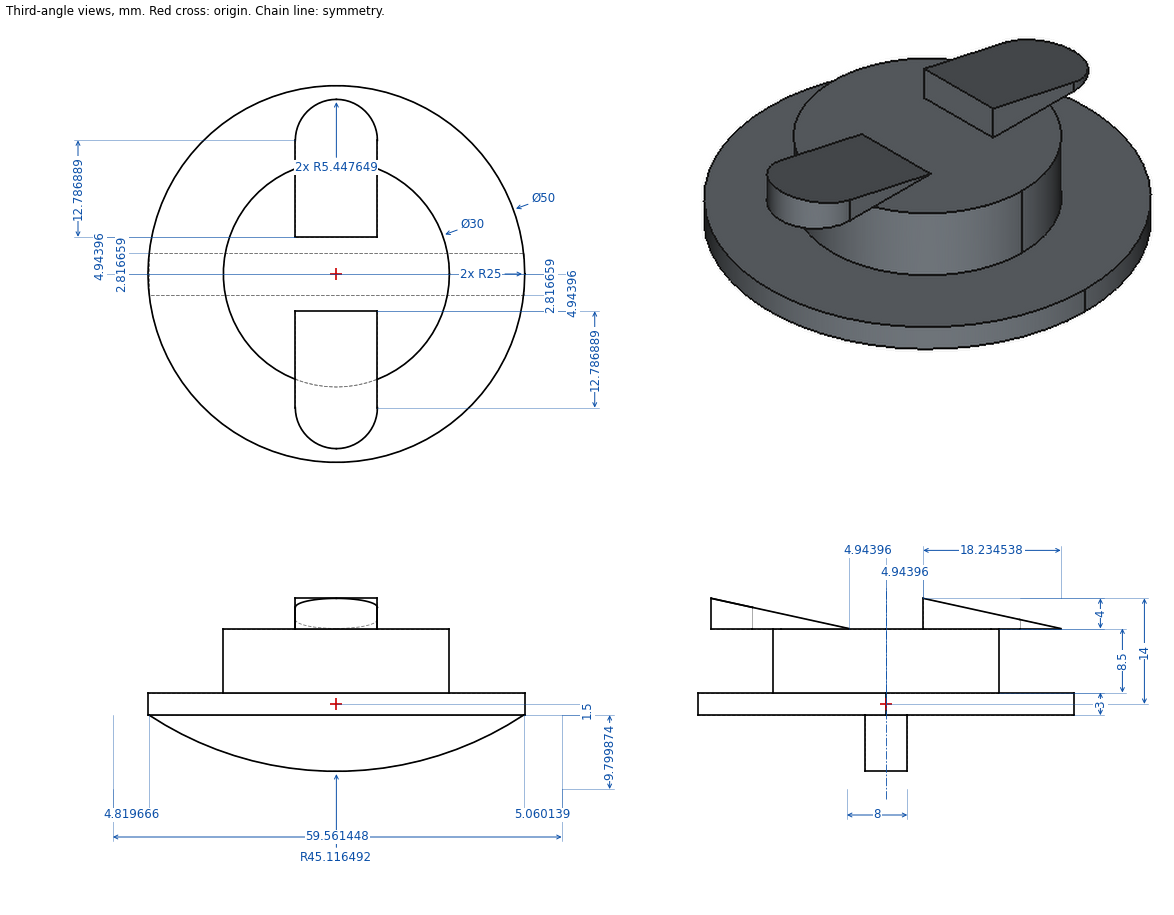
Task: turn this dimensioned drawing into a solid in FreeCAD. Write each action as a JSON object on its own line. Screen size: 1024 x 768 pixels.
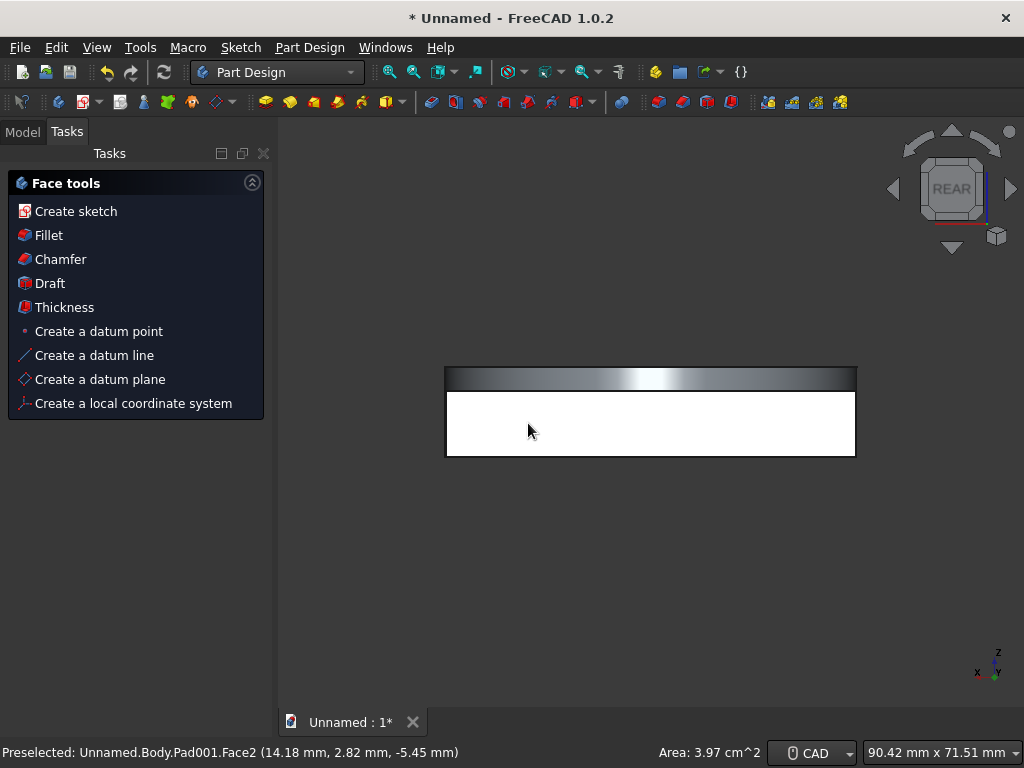
{"action": "left_click", "coordinate": [84, 102]}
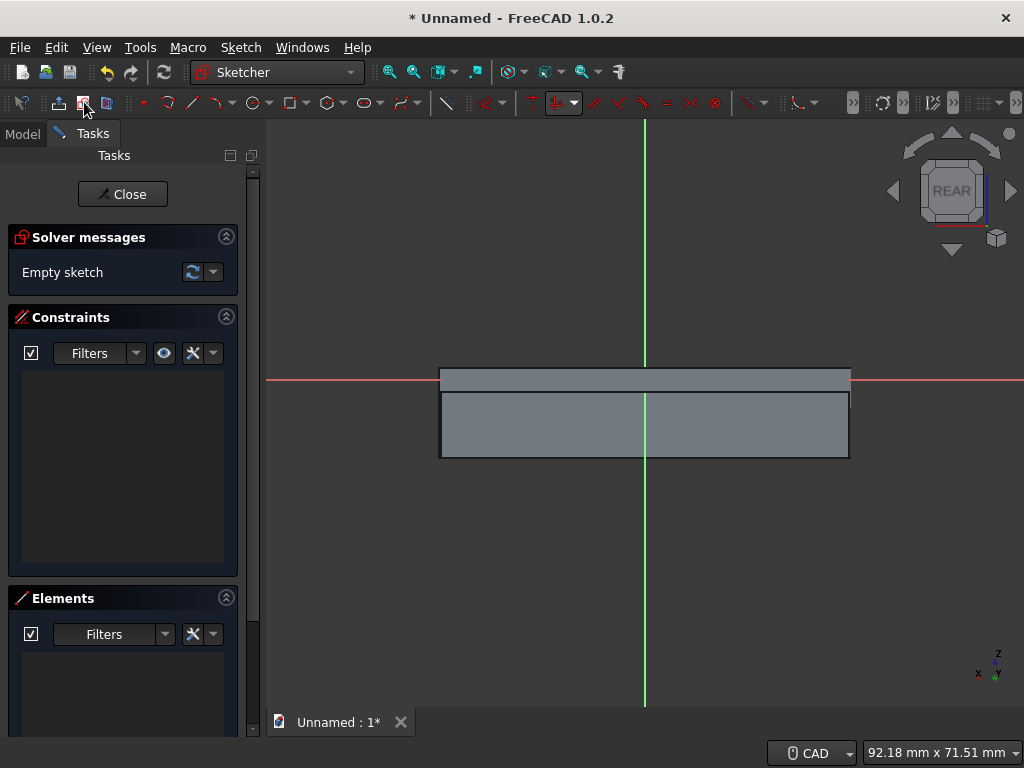
{"action": "left_click", "coordinate": [108, 104]}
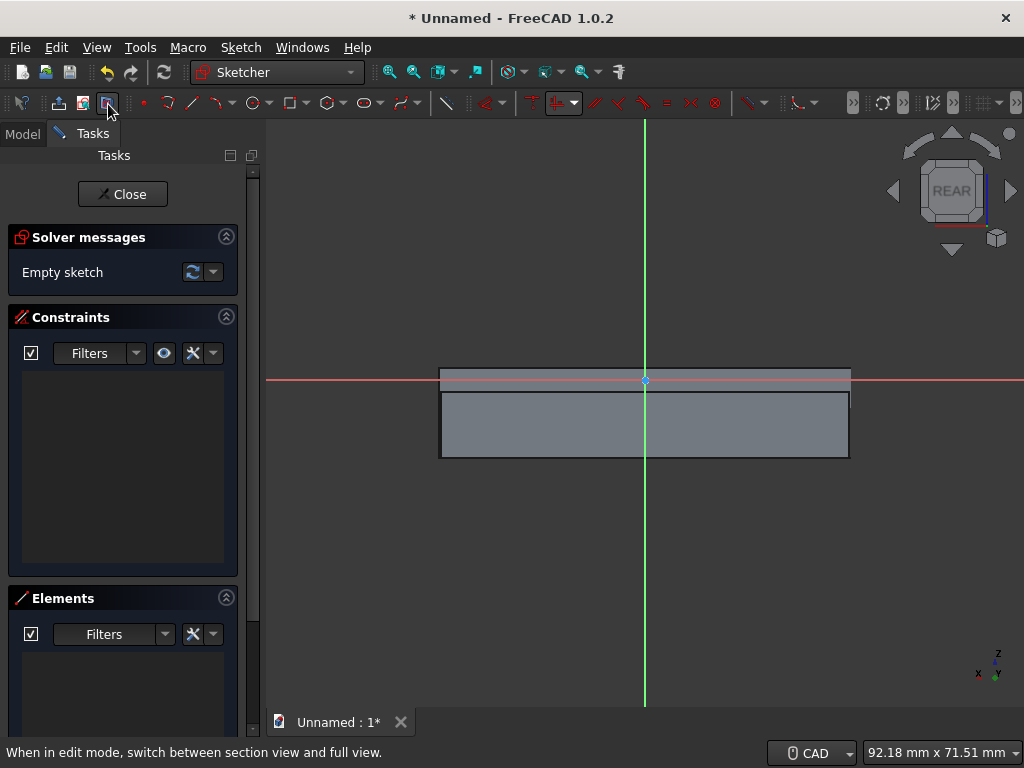
{"action": "scroll", "coordinate": [294, 352], "scroll_direction": "down", "scroll_amount": 1}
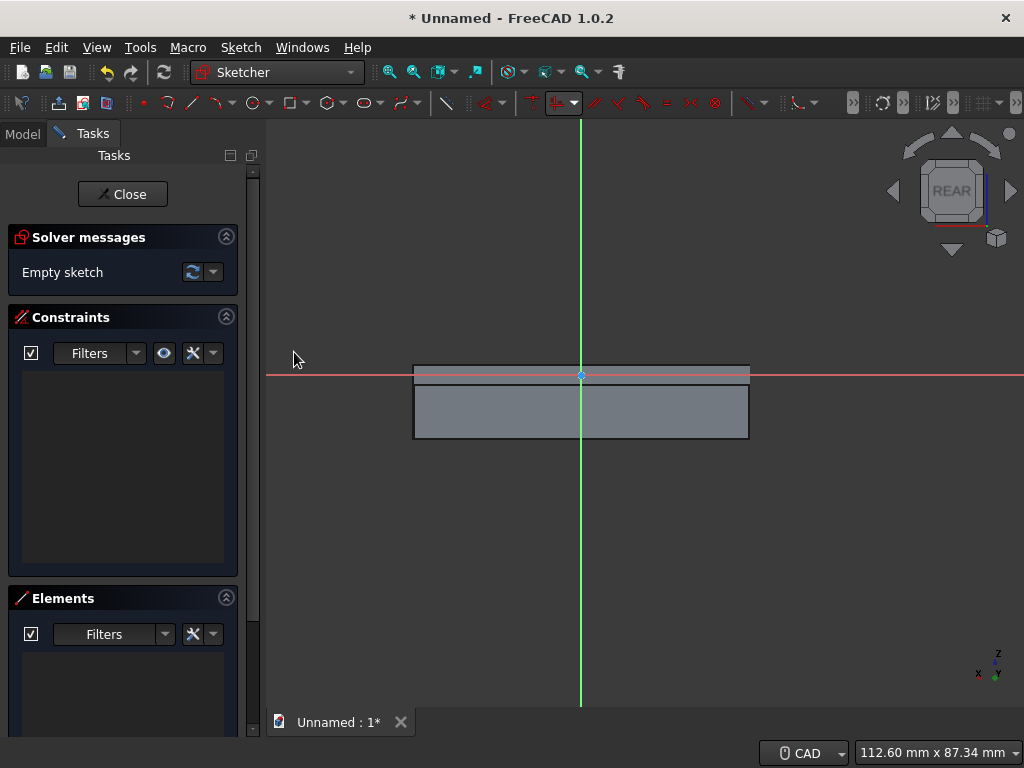
{"action": "left_click", "coordinate": [168, 104]}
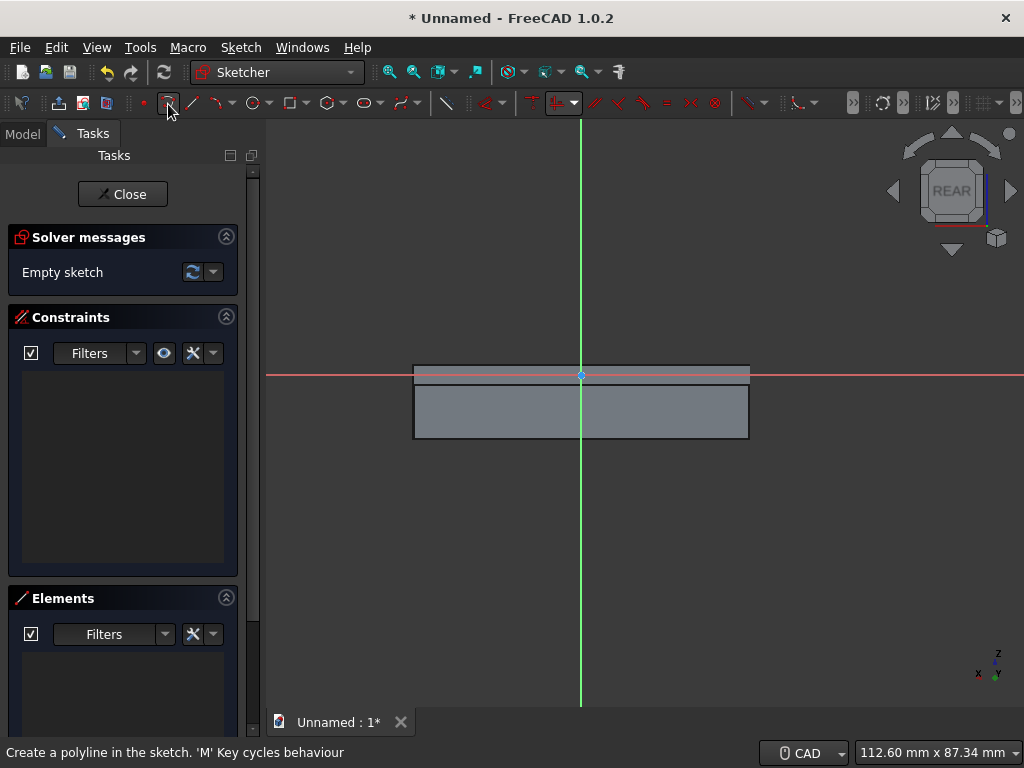
{"action": "scroll", "coordinate": [414, 385], "scroll_direction": "up", "scroll_amount": 3}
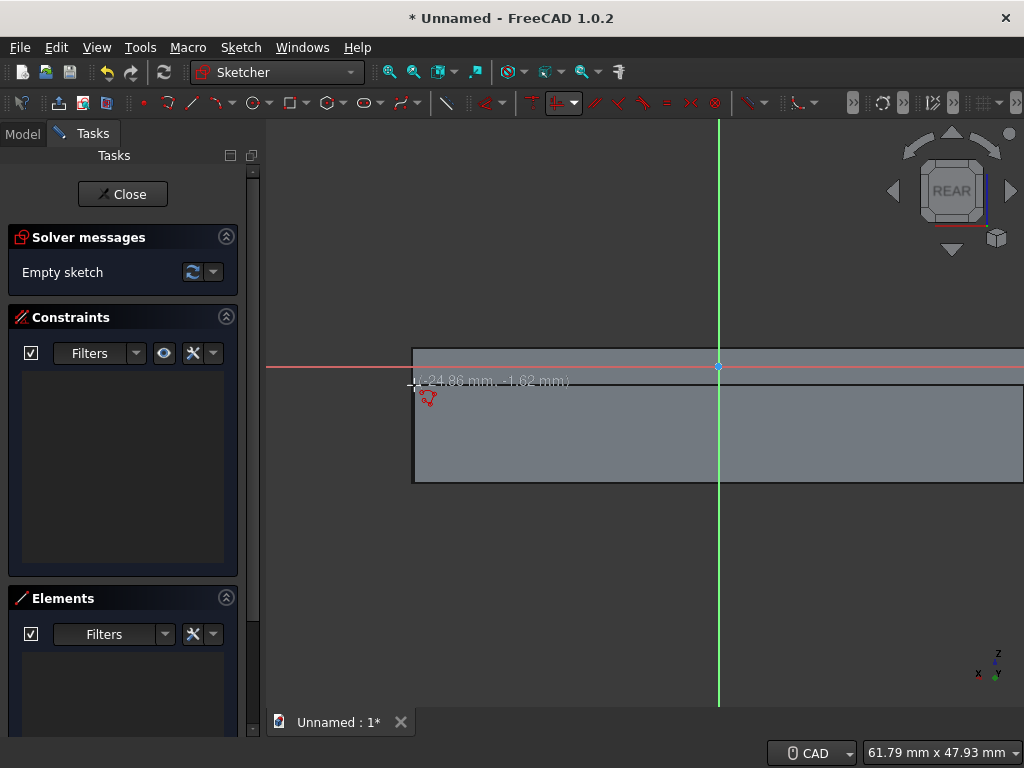
{"action": "left_click", "coordinate": [414, 385]}
{"action": "left_click", "coordinate": [352, 385]}
{"action": "left_click", "coordinate": [352, 505]}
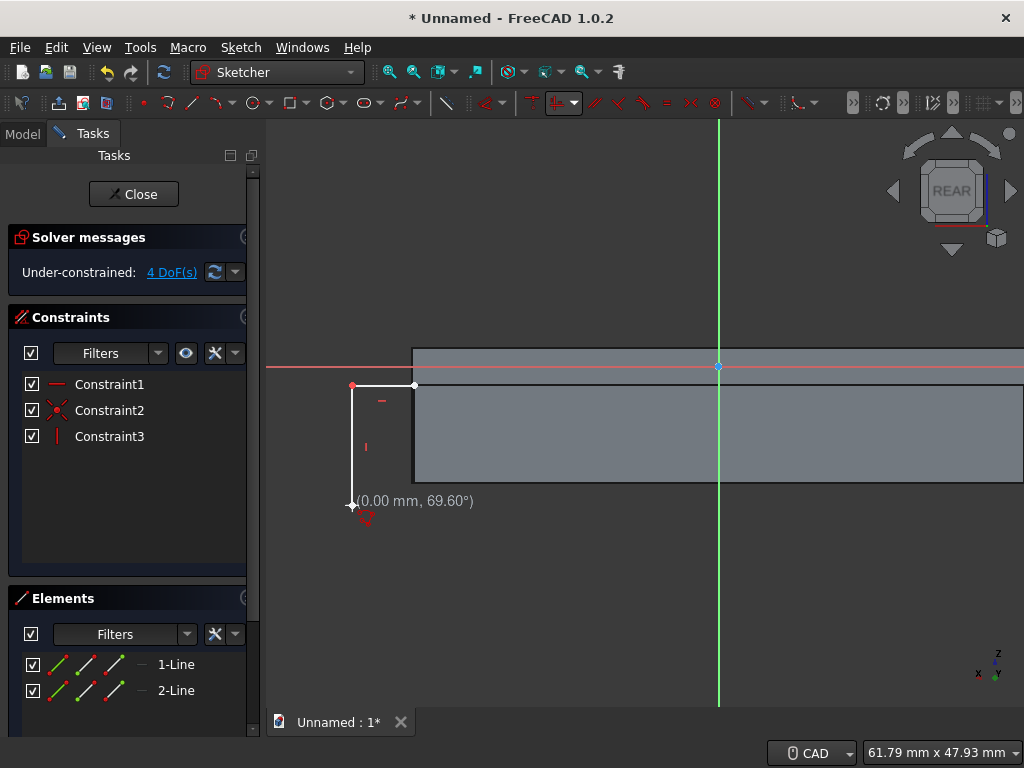
{"action": "scroll", "coordinate": [405, 385], "scroll_direction": "down", "scroll_amount": 3}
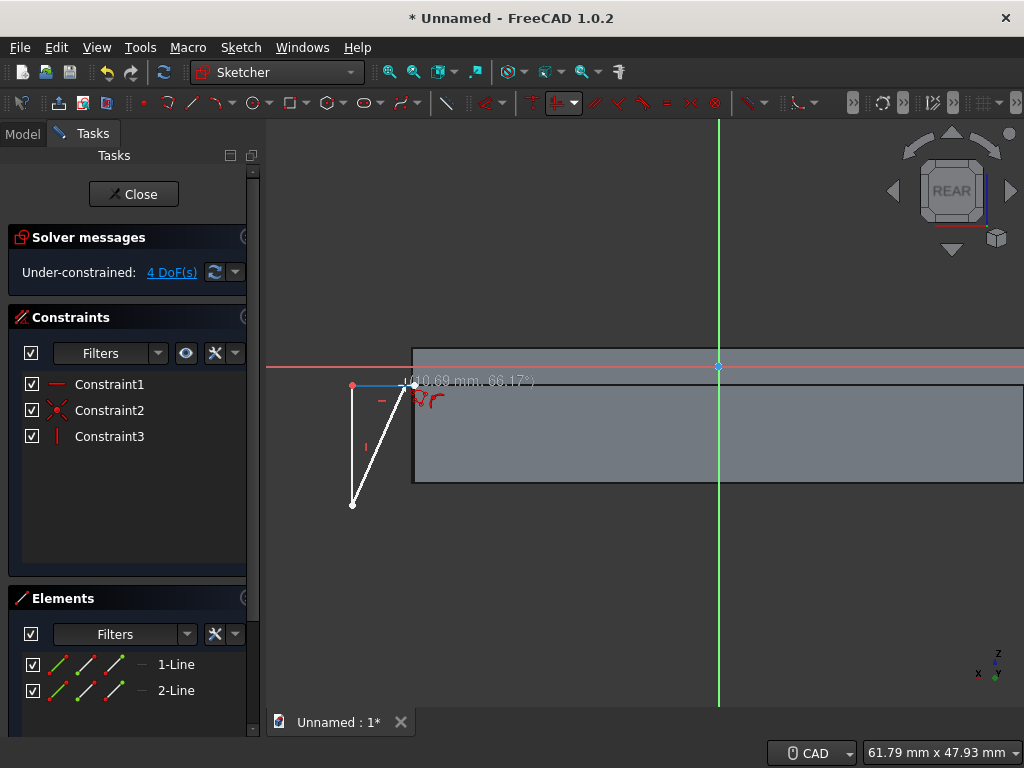
{"action": "left_click", "coordinate": [777, 451]}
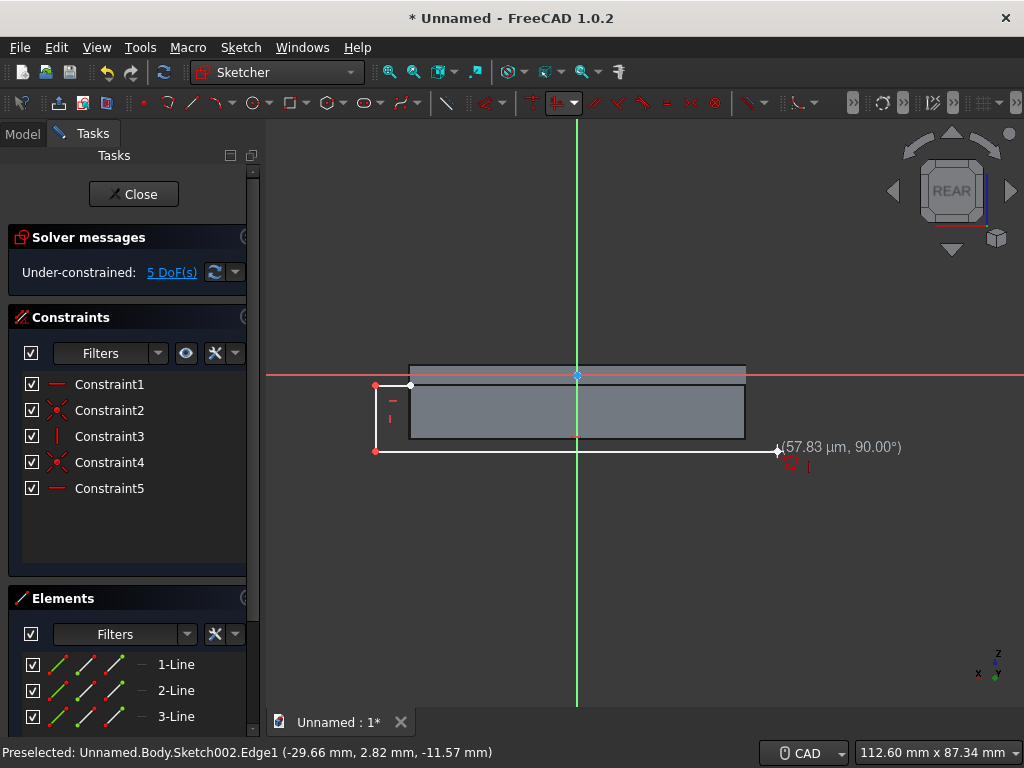
{"action": "scroll", "coordinate": [777, 385], "scroll_direction": "up", "scroll_amount": 3}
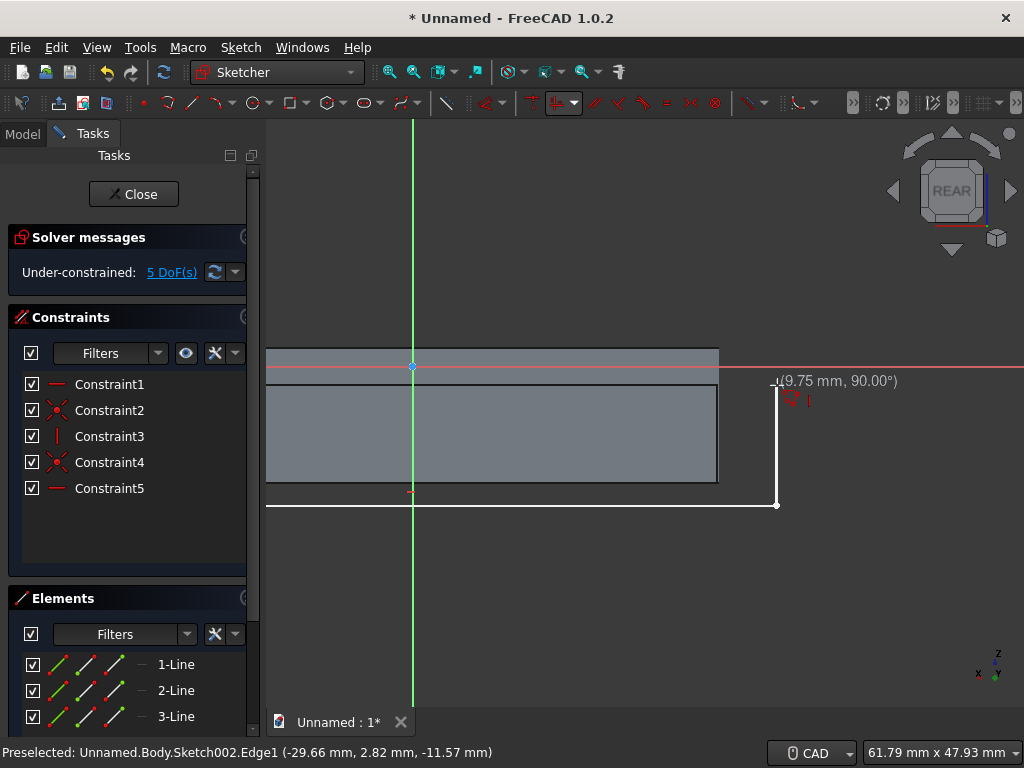
{"action": "left_click", "coordinate": [776, 385]}
{"action": "left_click", "coordinate": [717, 385]}
{"action": "right_click", "coordinate": [717, 385]}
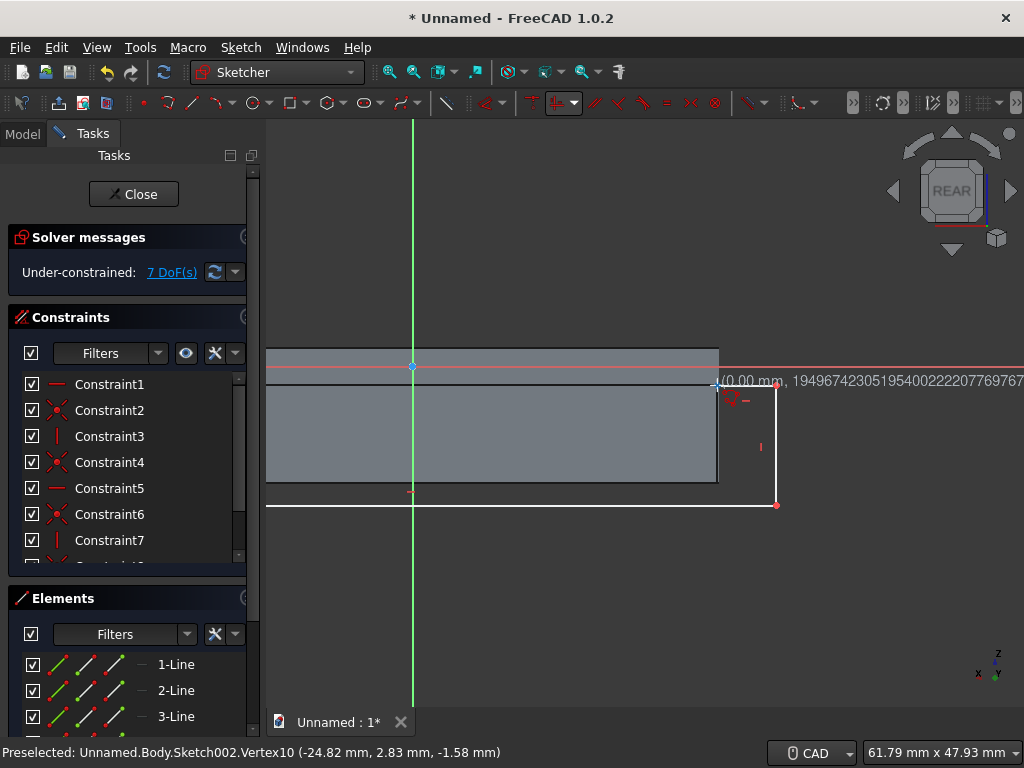
{"action": "left_click", "coordinate": [216, 104]}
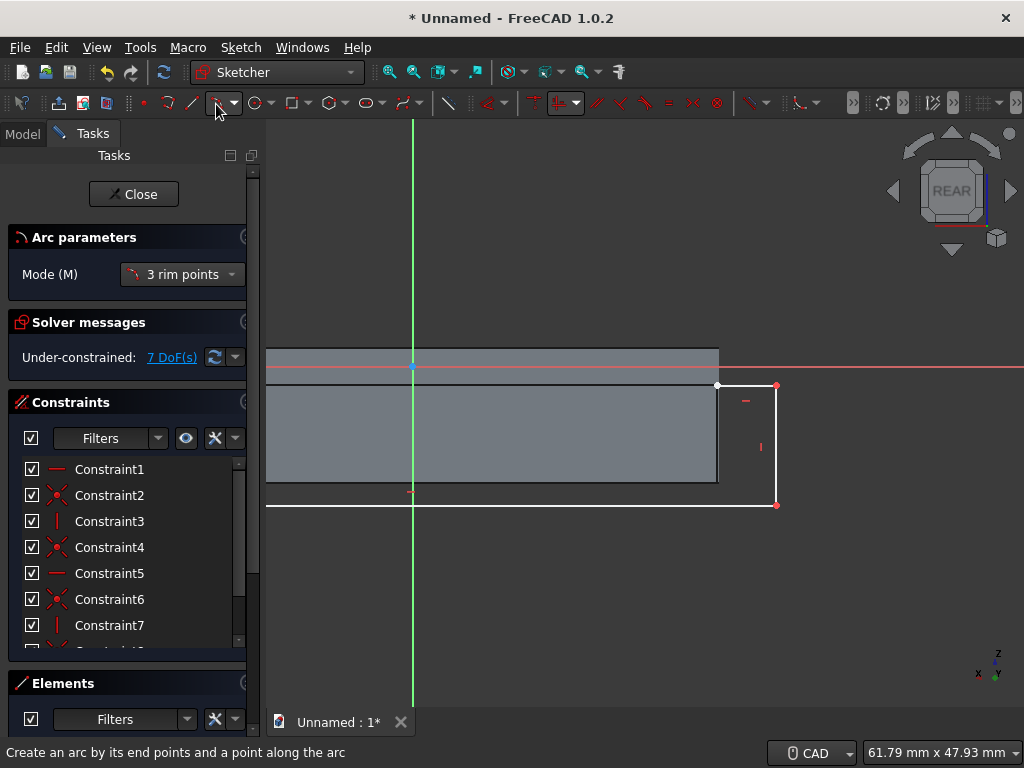
{"action": "left_click", "coordinate": [717, 386]}